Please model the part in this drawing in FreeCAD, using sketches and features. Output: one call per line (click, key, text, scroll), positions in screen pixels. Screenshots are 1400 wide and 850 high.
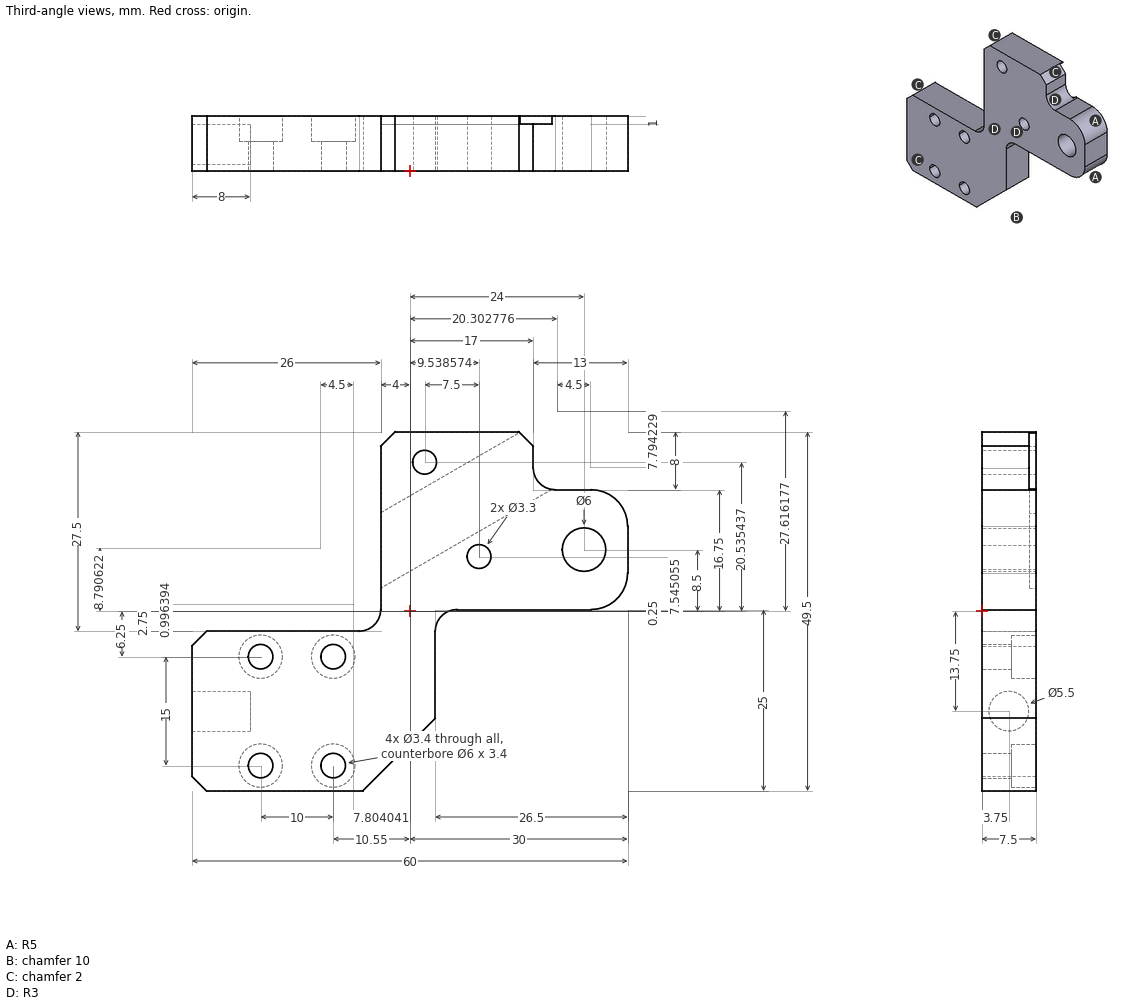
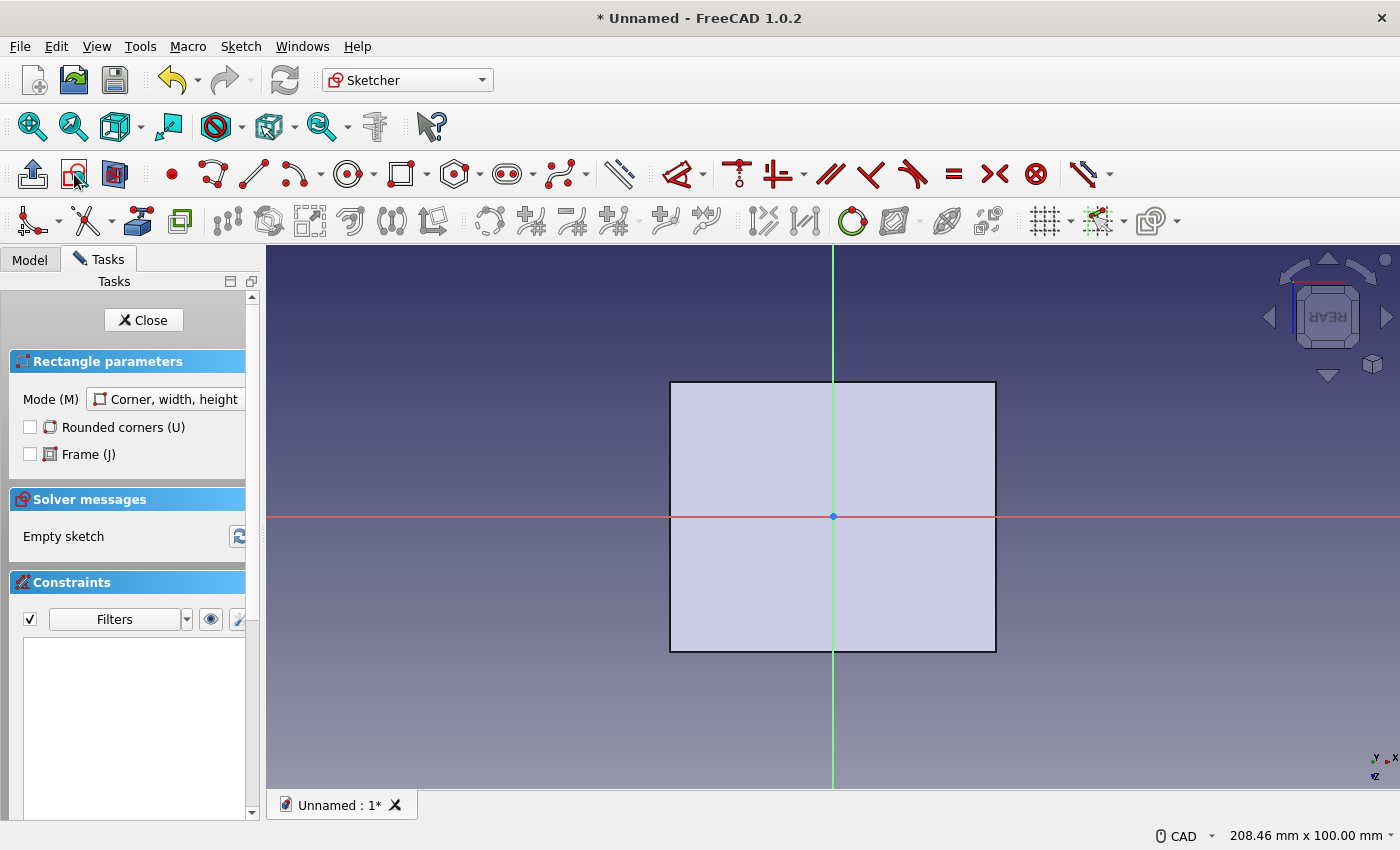
click(852, 382)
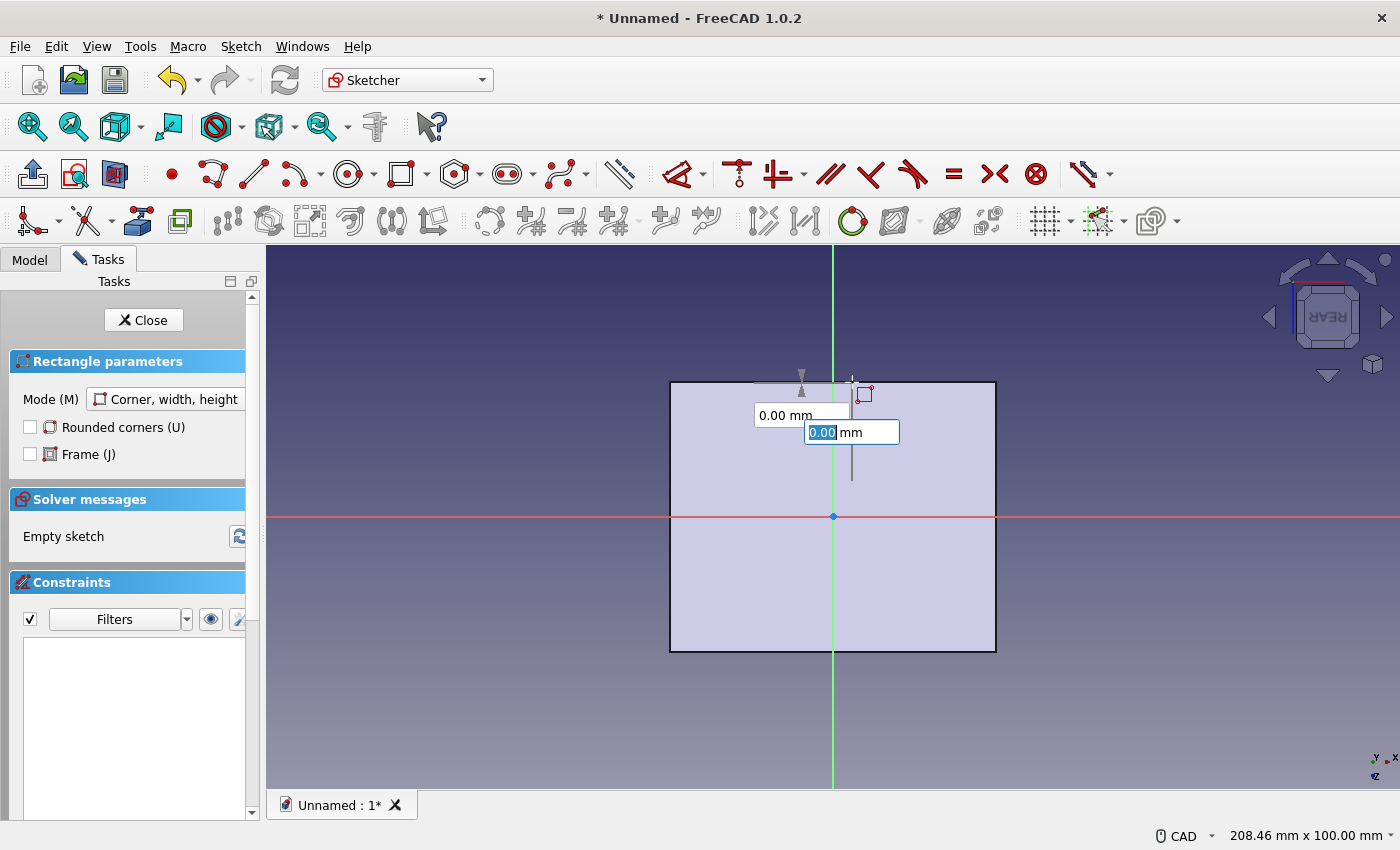
scroll(996, 518, up, 13)
move(991, 517)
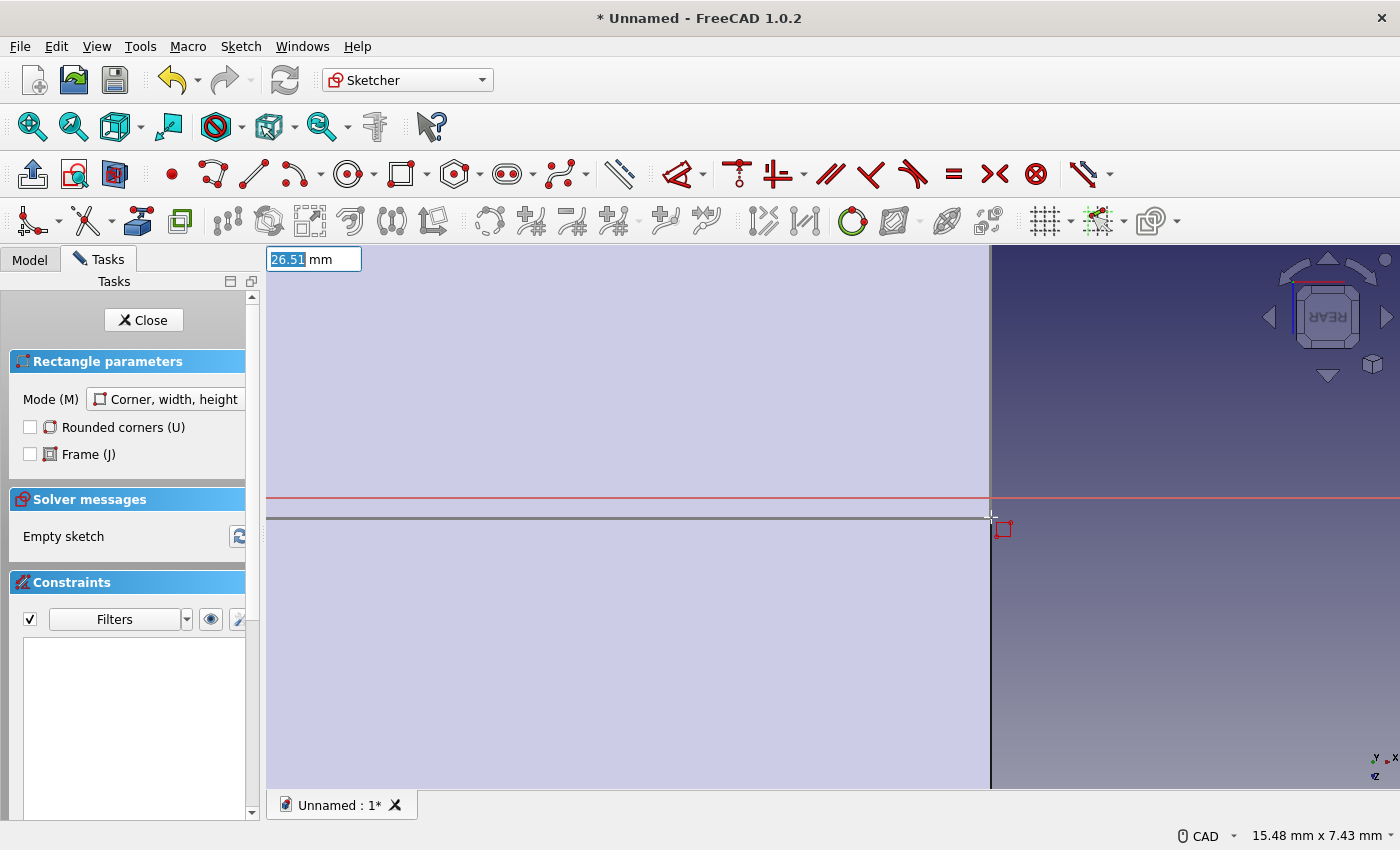
text(26.5)
key(Tab)
text(25)
key(Return)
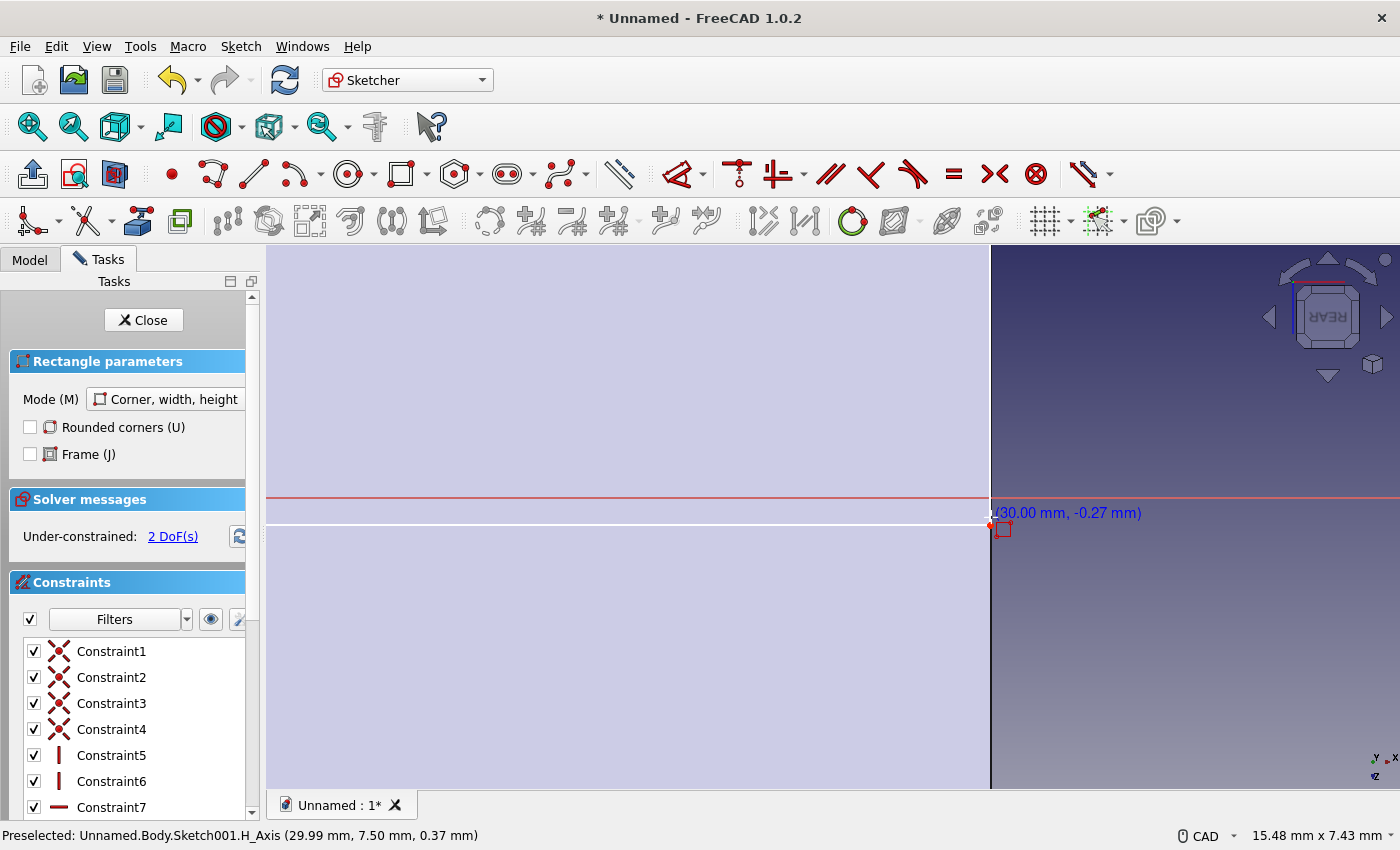
scroll(961, 519, down, 12)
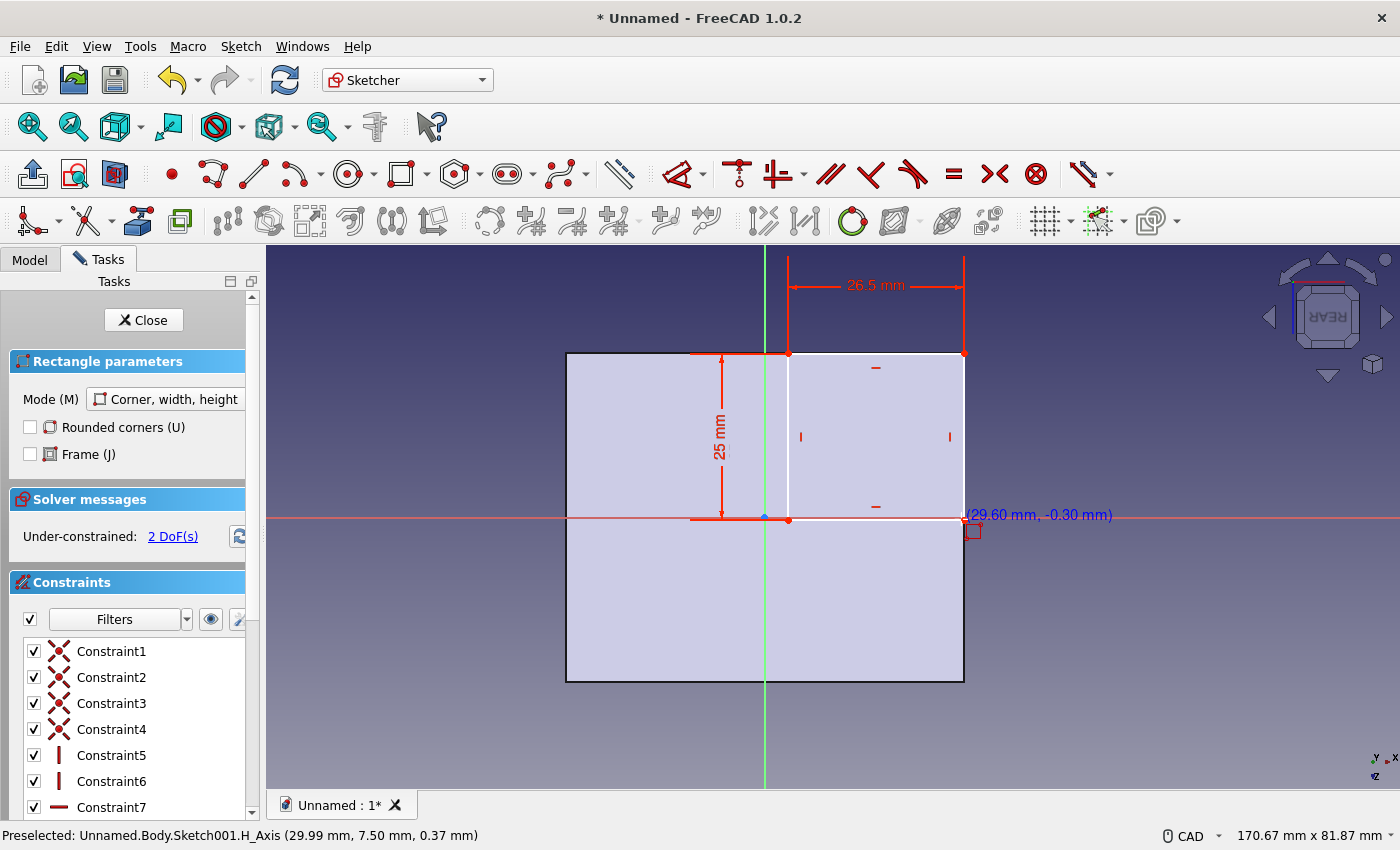
click(878, 629)
move(964, 682)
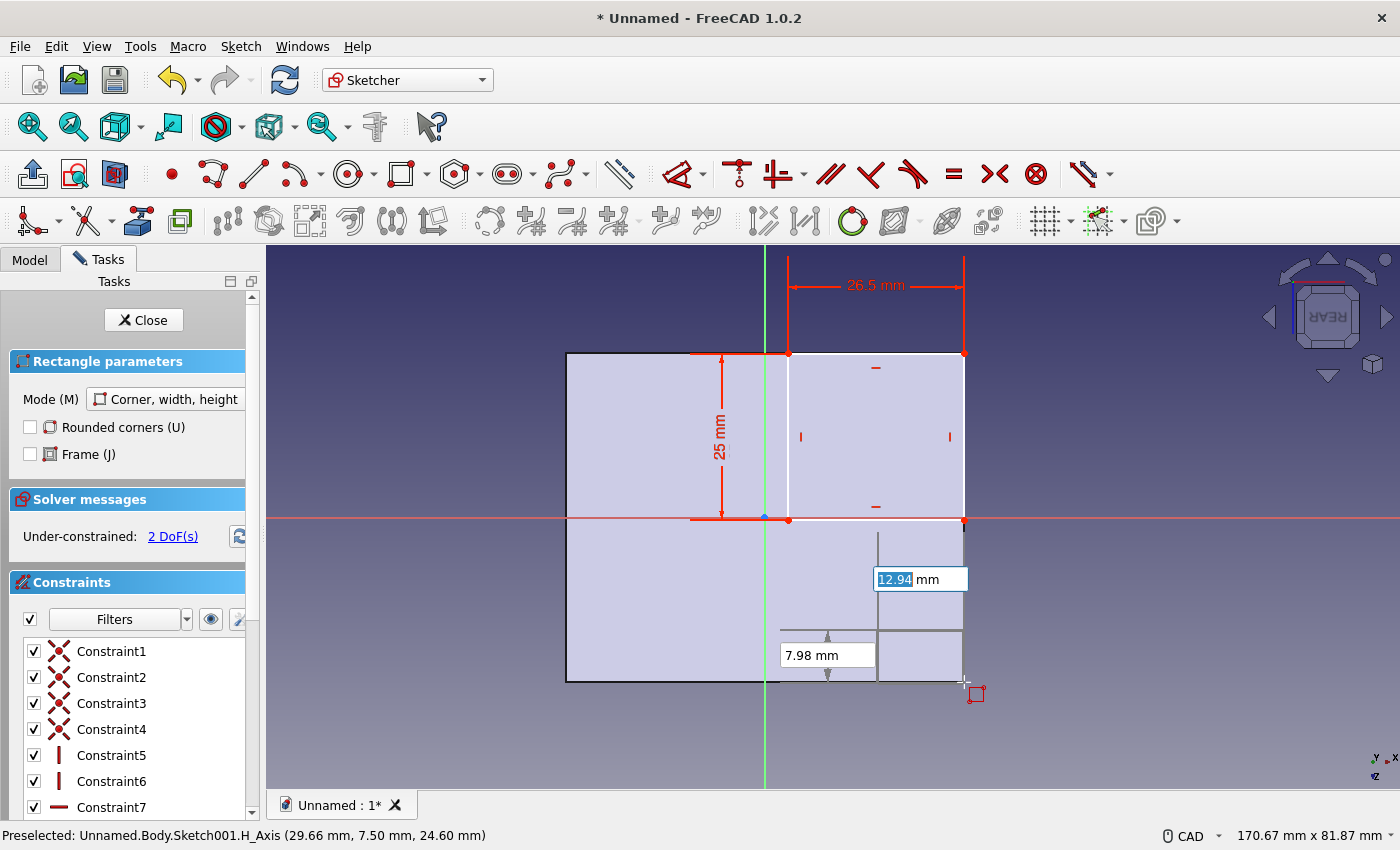
text(13)
key(Tab)
text(8)
key(Return)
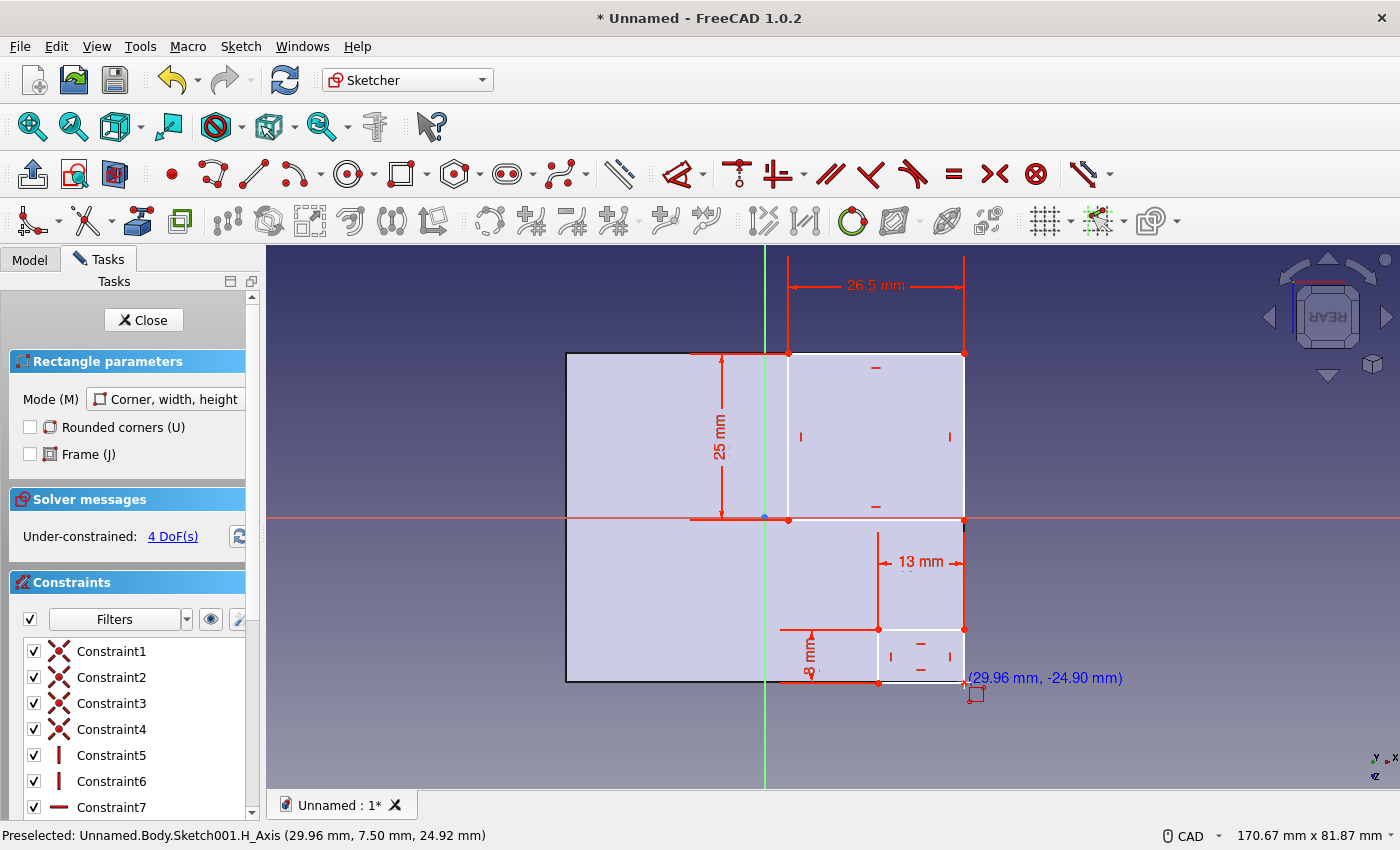
click(566, 499)
move(738, 682)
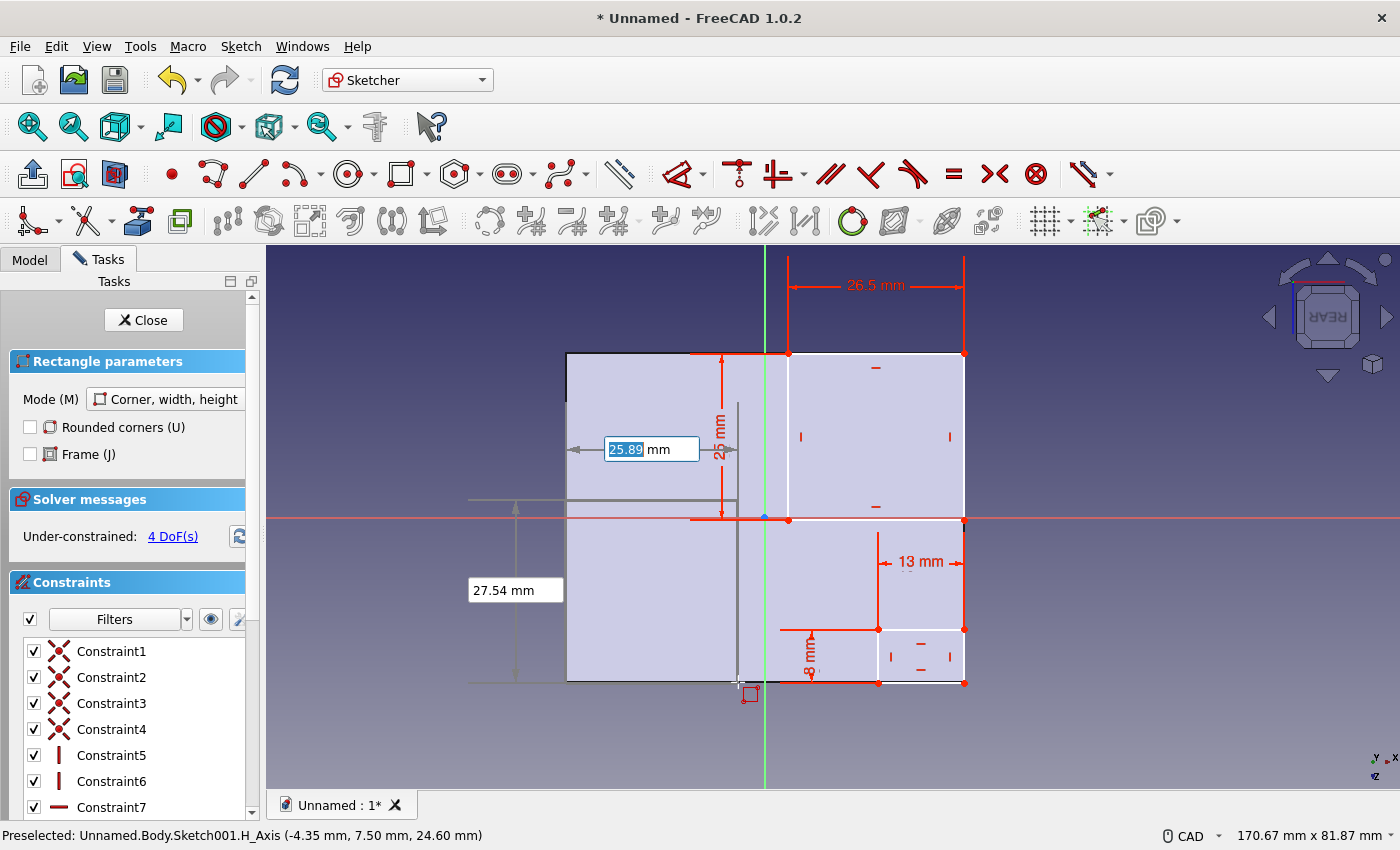
text(26)
key(Tab)
text(27.5)
key(Return)
key(Escape)